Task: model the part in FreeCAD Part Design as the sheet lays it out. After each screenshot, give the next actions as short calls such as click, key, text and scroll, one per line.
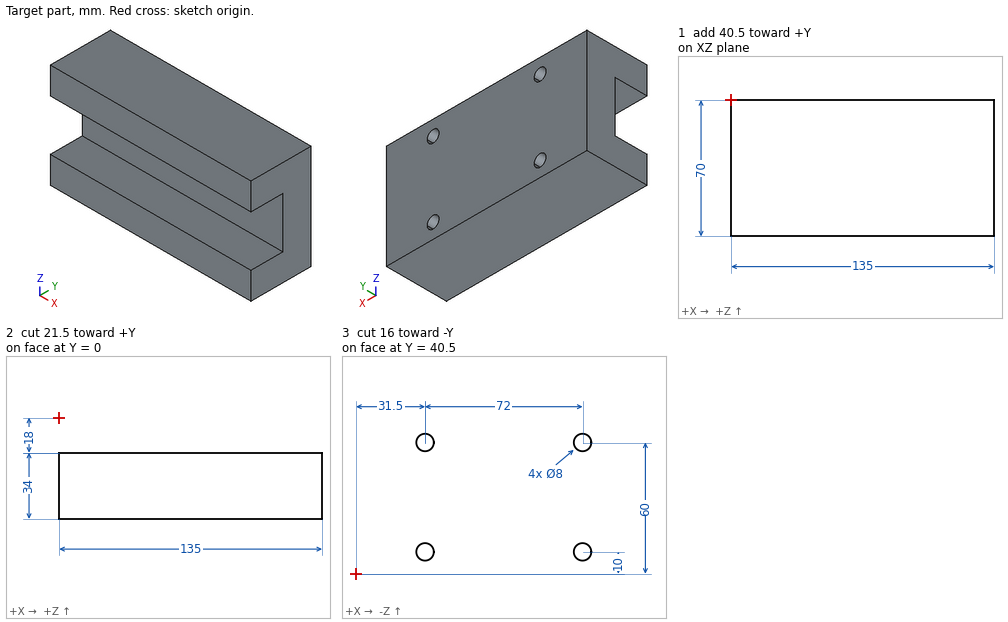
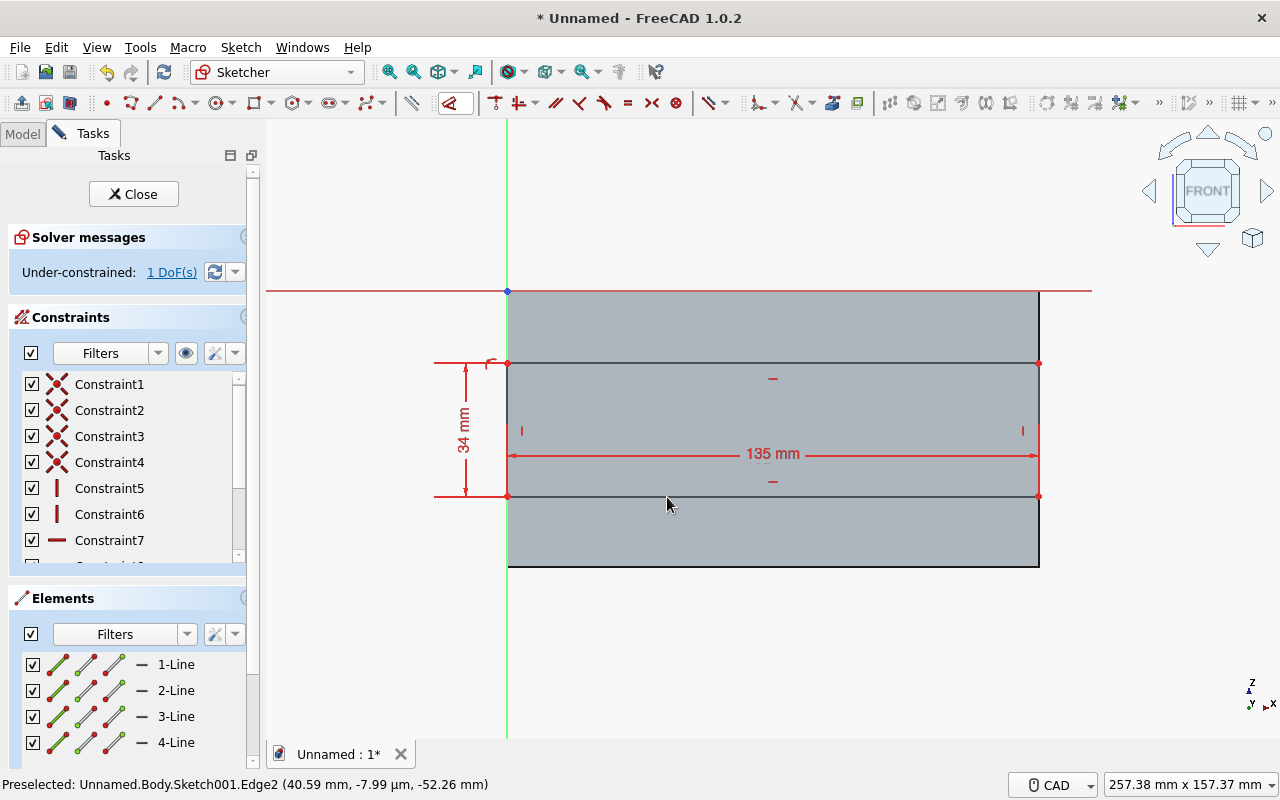
click(507, 363)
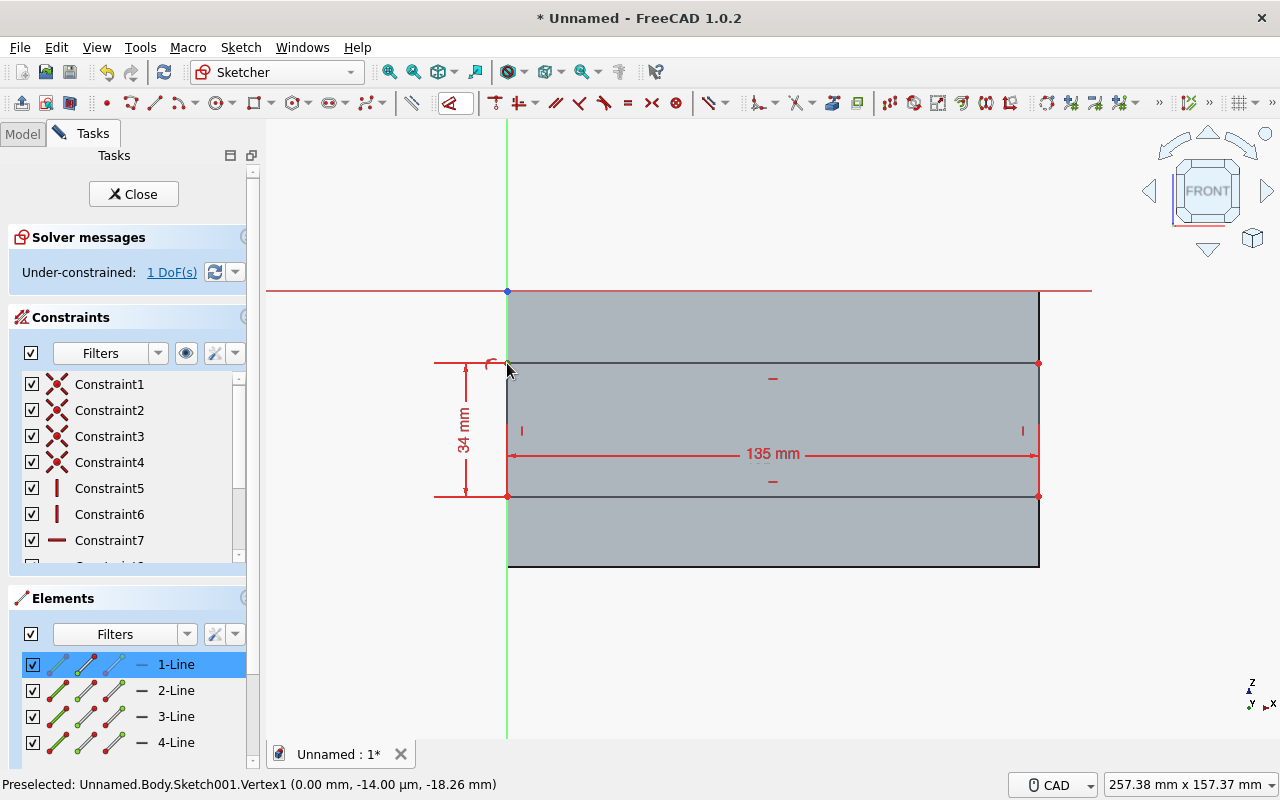
click(468, 104)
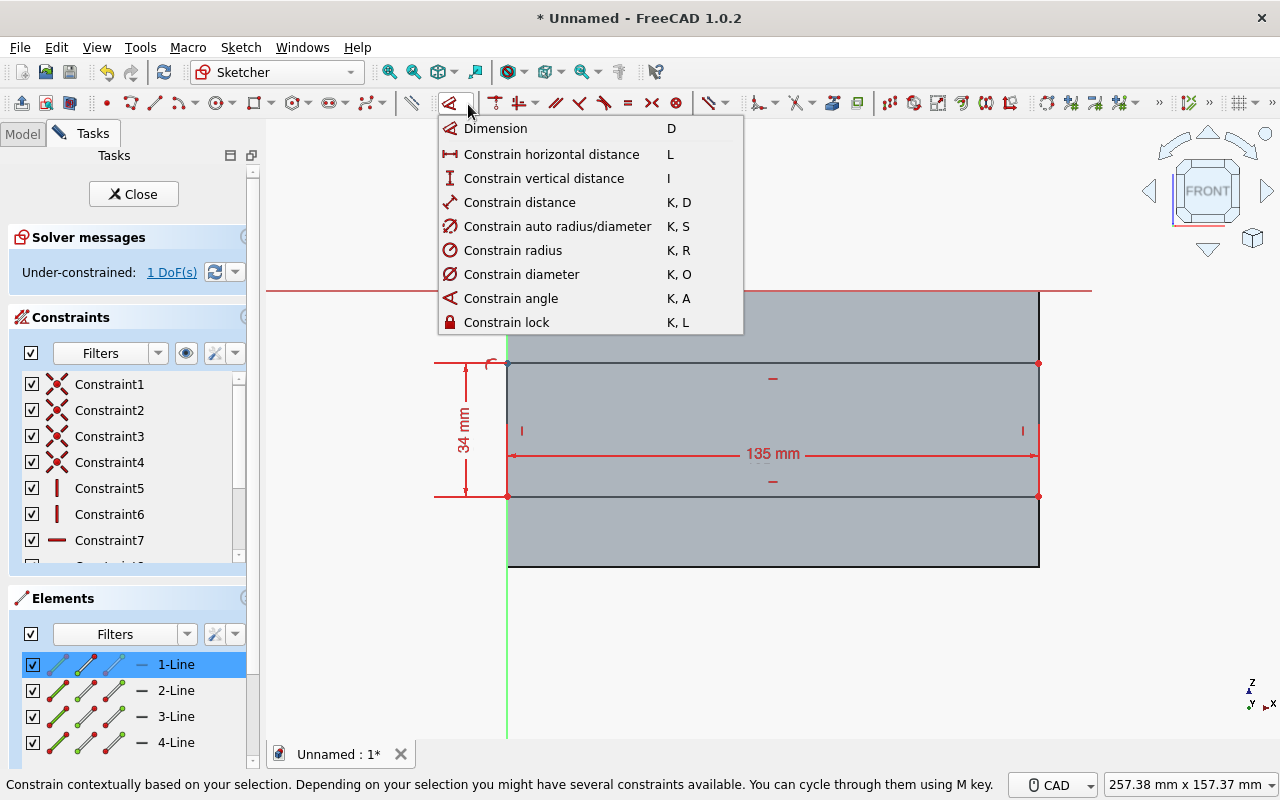
click(591, 178)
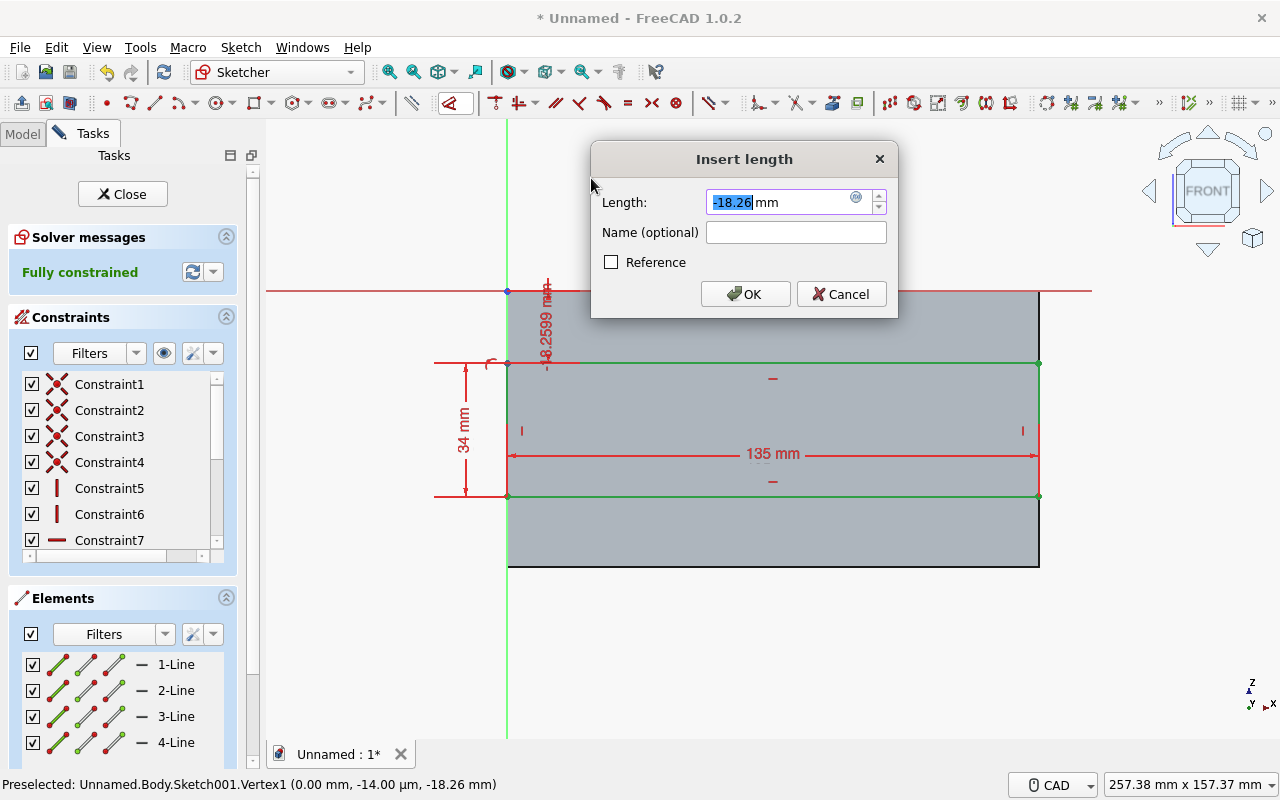
text(-18)
key(Return)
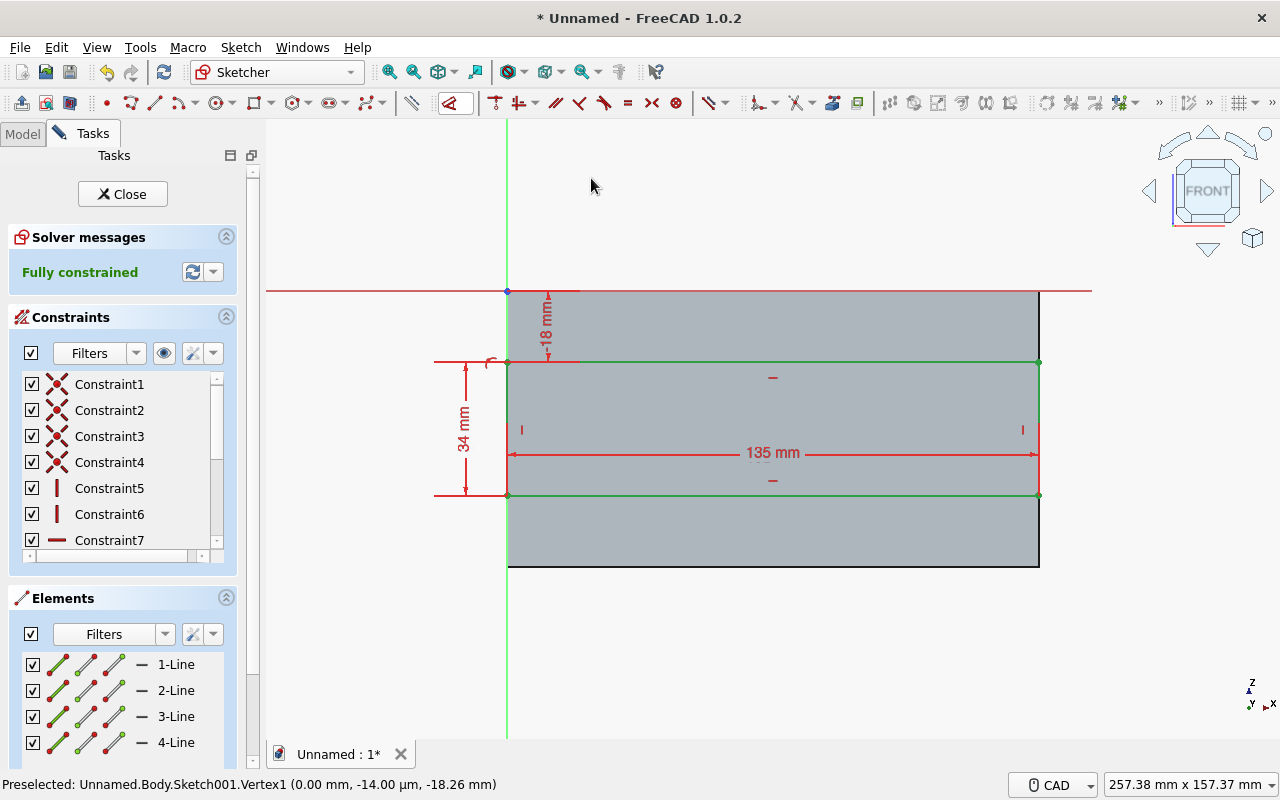
click(123, 194)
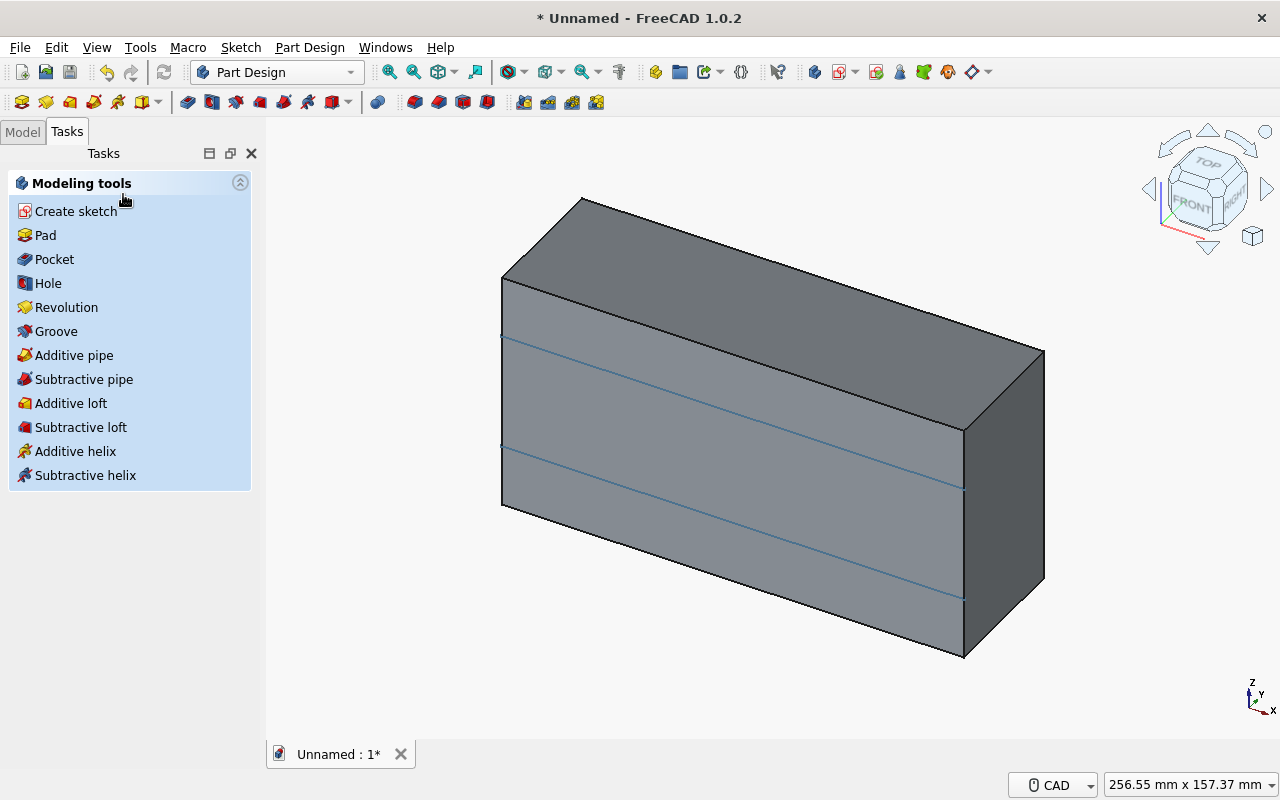
click(188, 102)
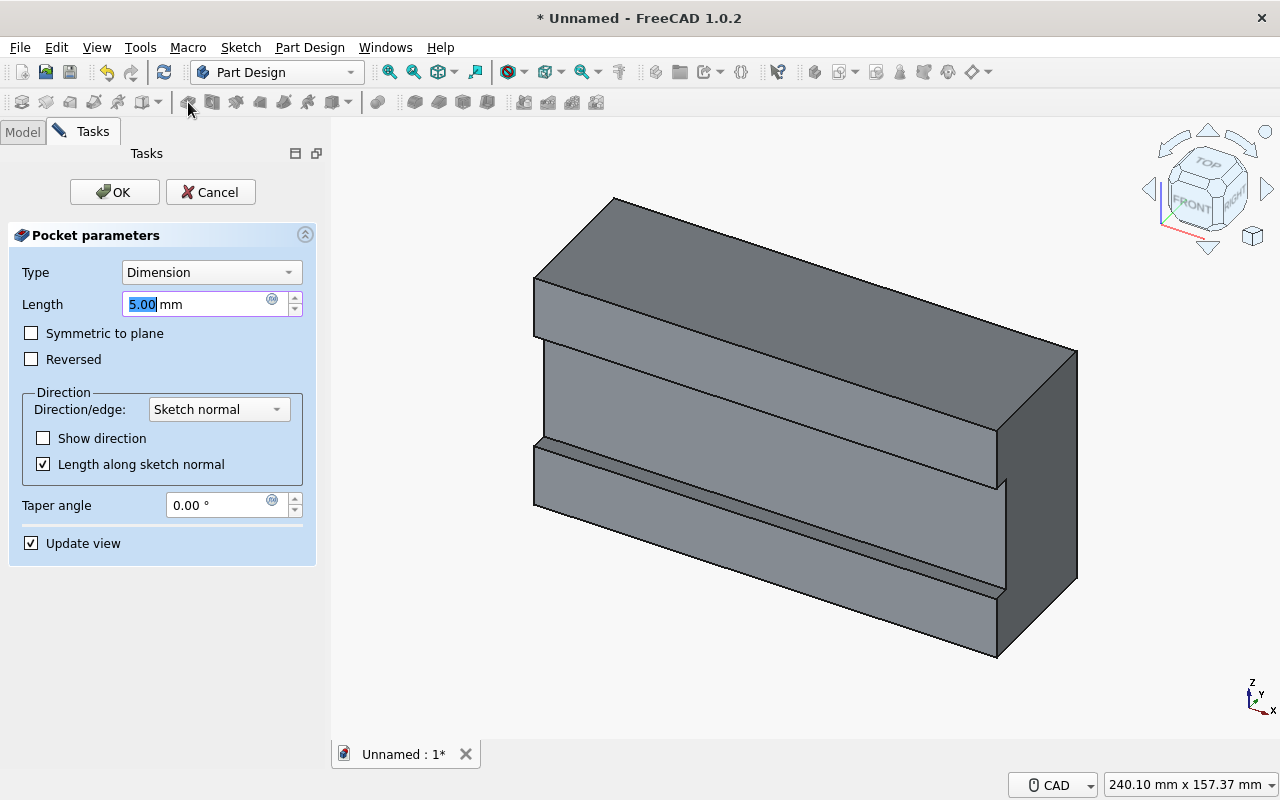
text(21.5)
key(Tab)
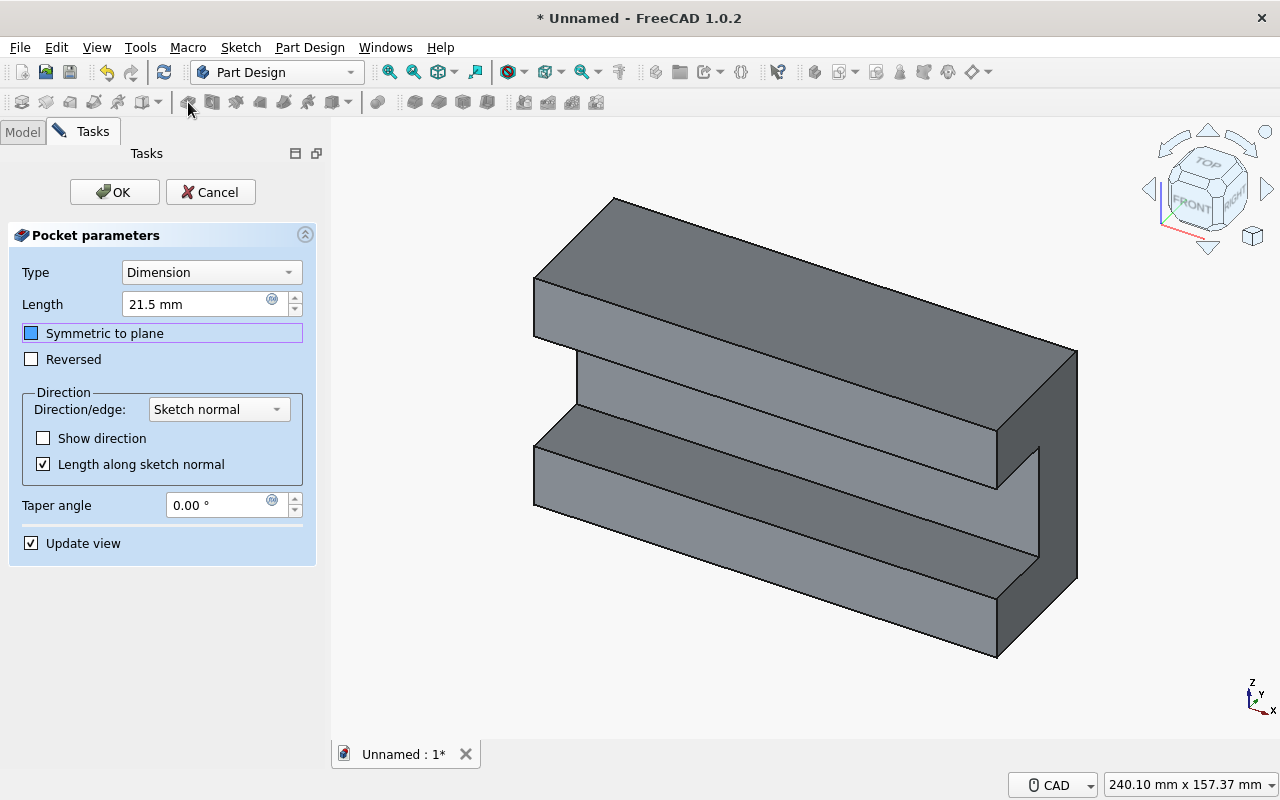
click(115, 192)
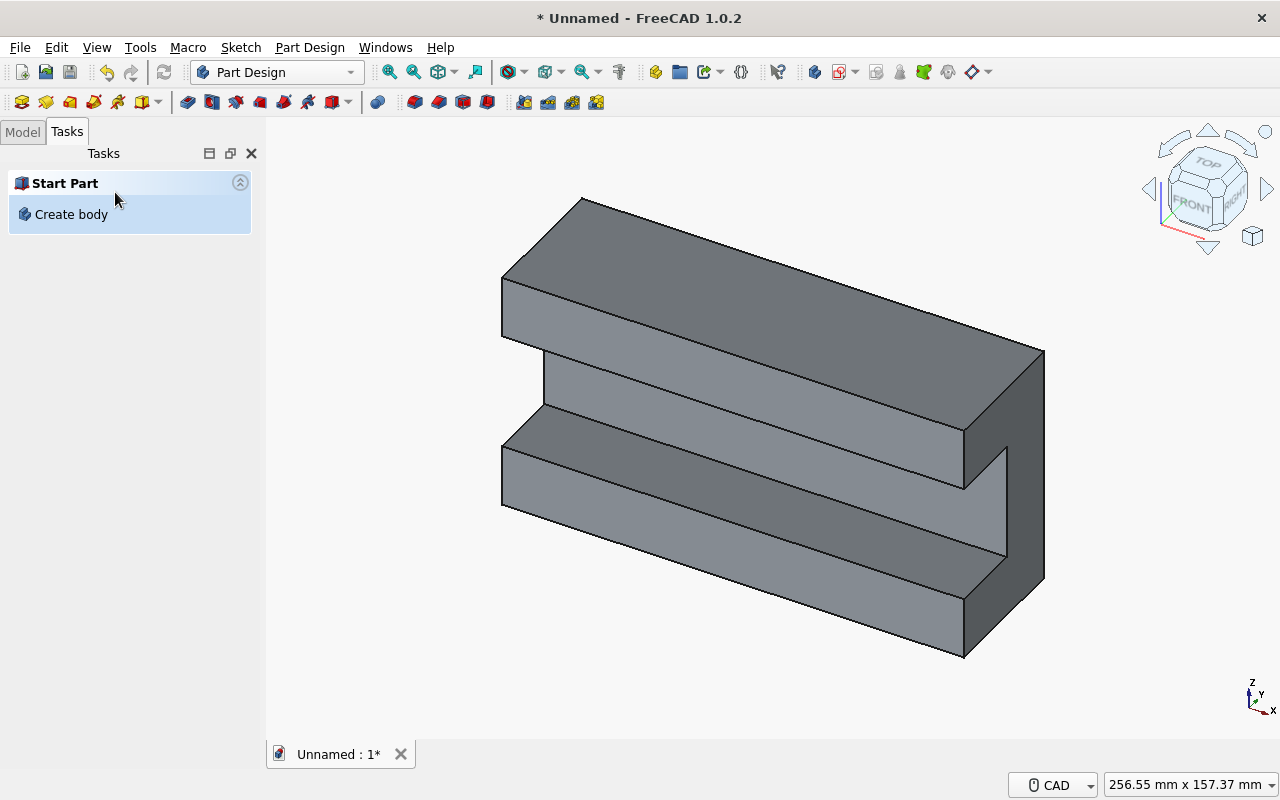
key(4)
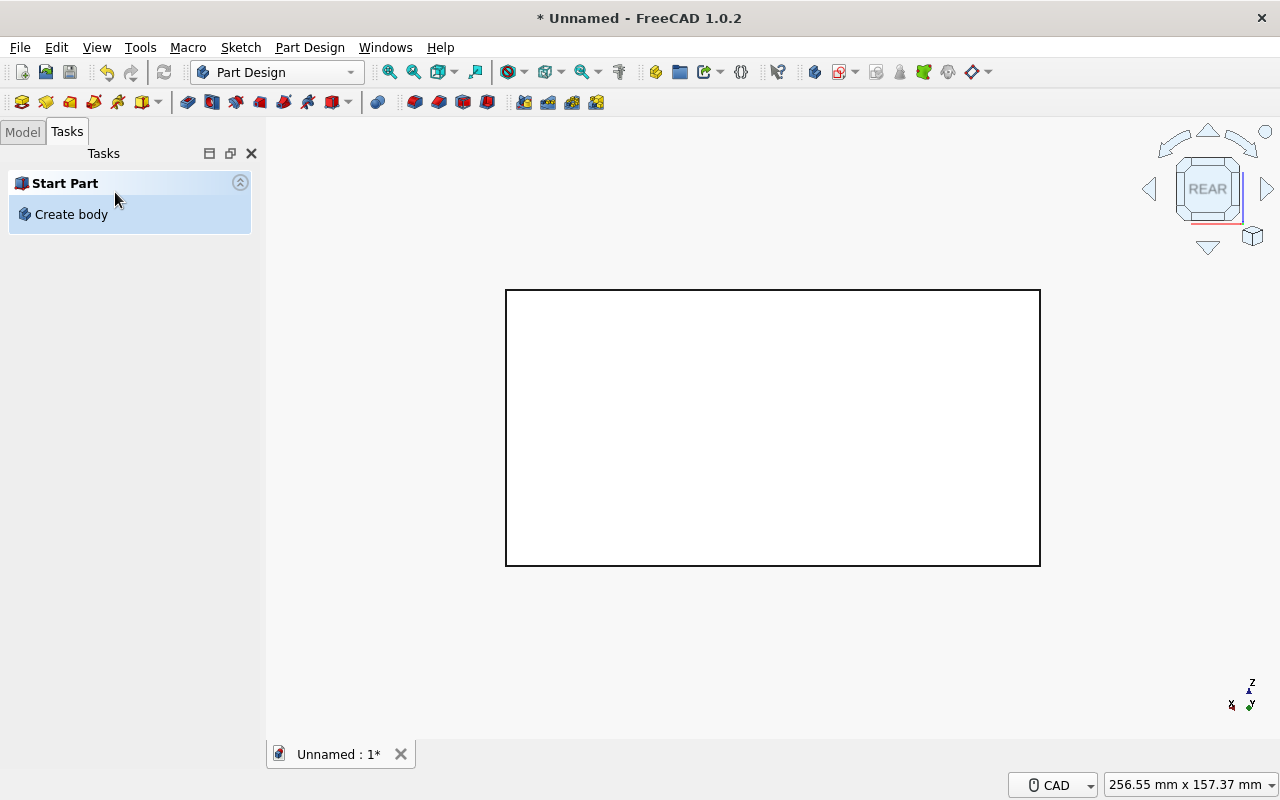
click(697, 427)